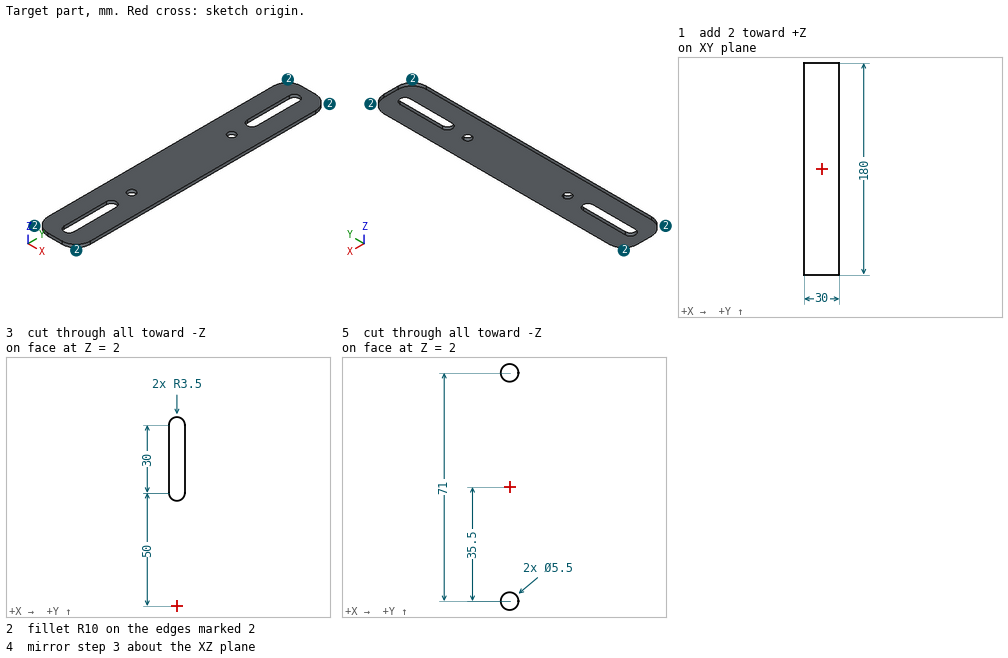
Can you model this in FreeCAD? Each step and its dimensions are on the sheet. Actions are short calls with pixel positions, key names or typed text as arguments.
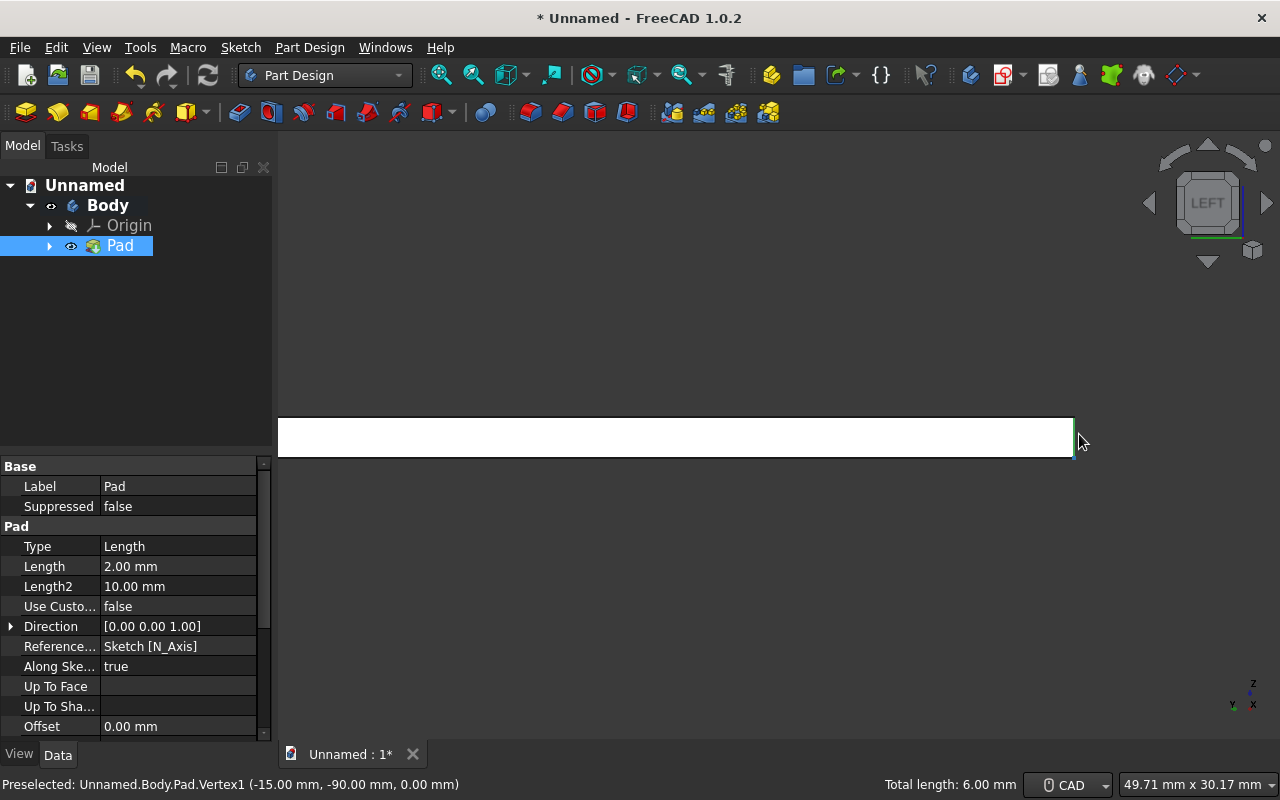
key(v)
key(f)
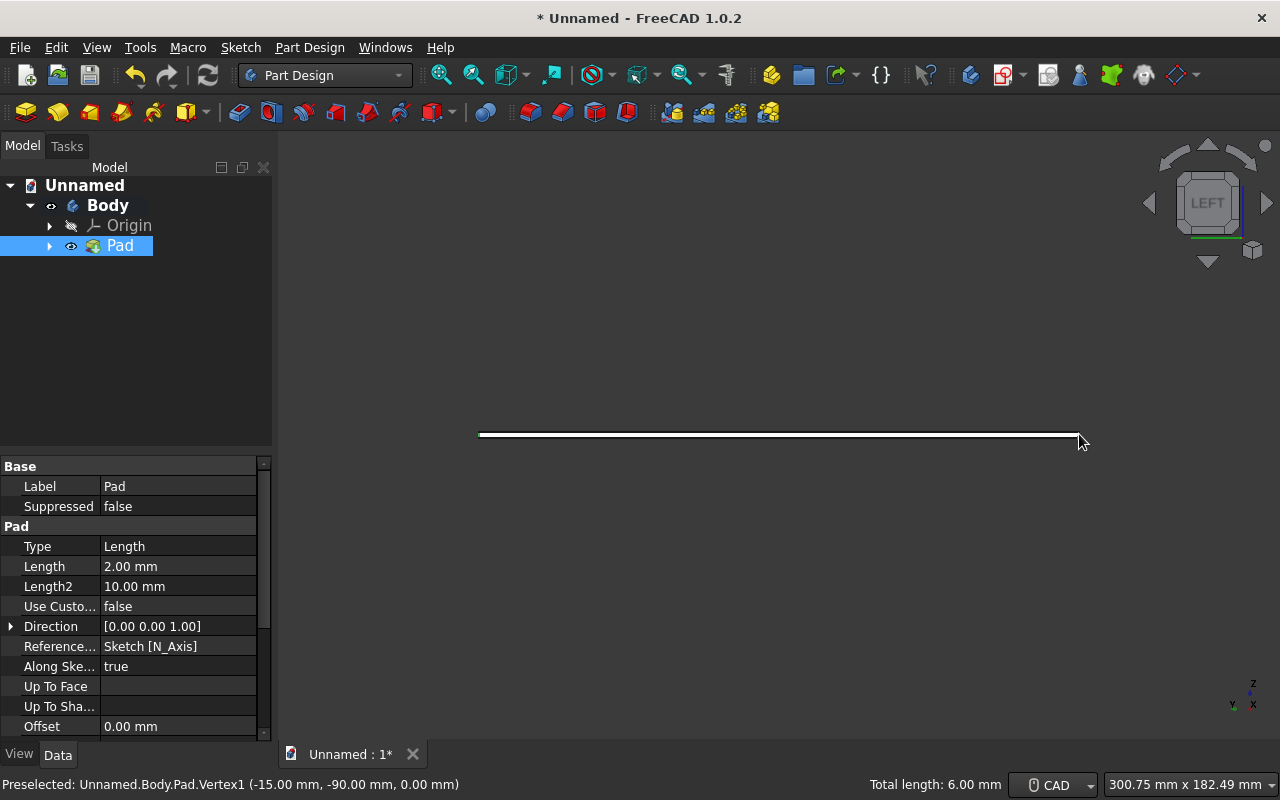
key(v)
key(3)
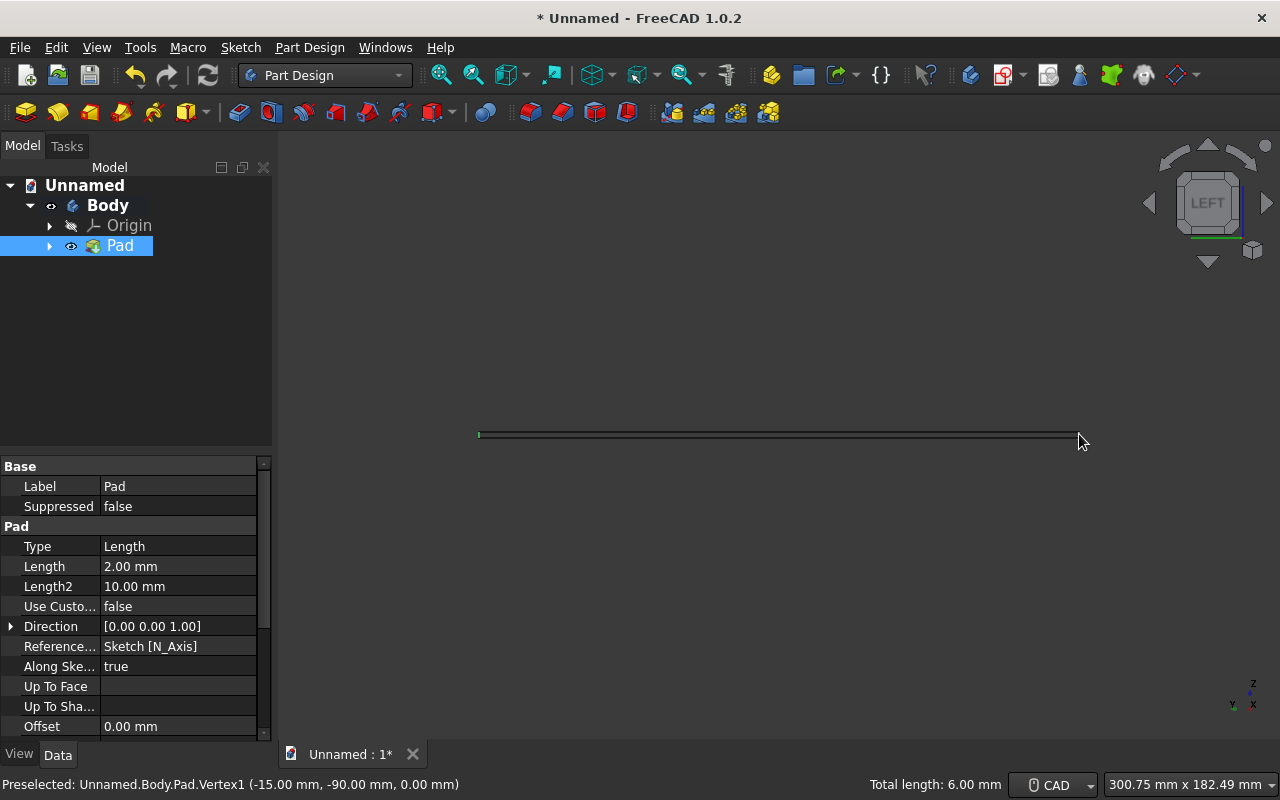
key(0)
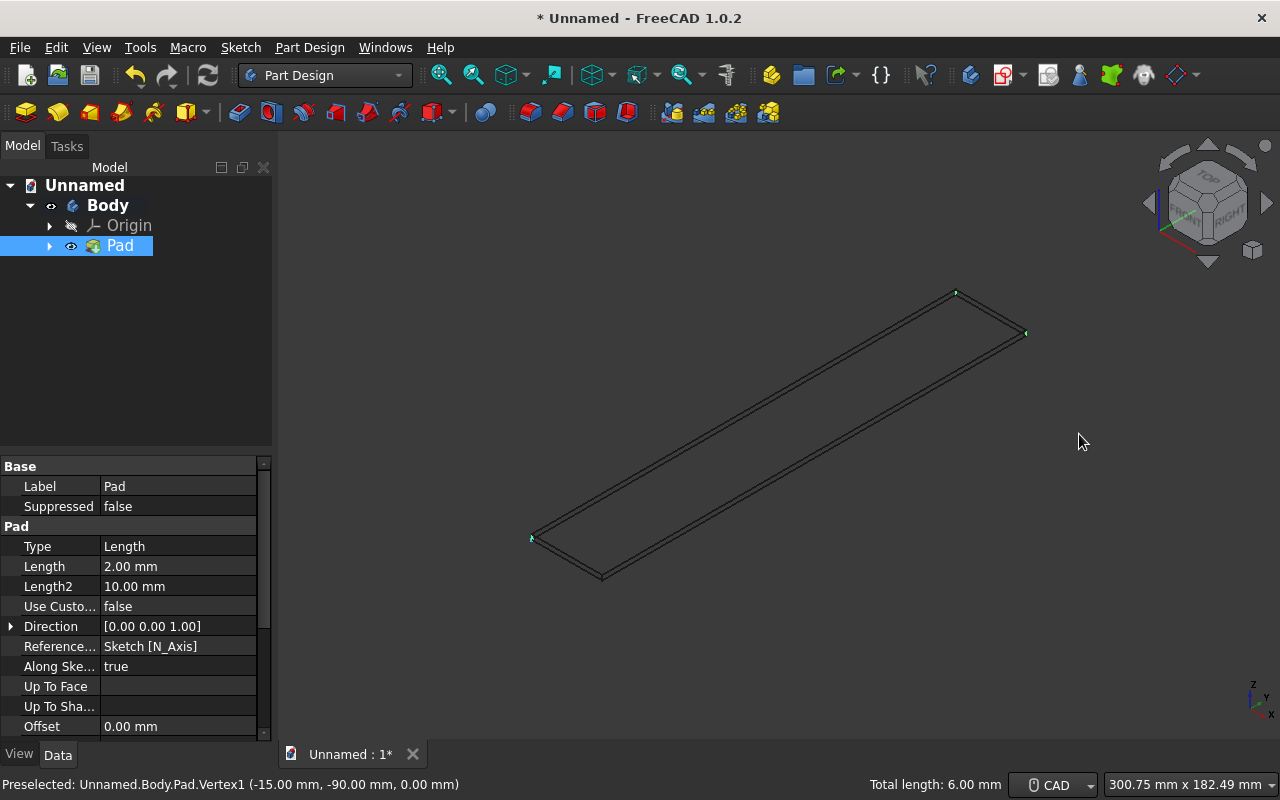
scroll(602, 577, up, 9)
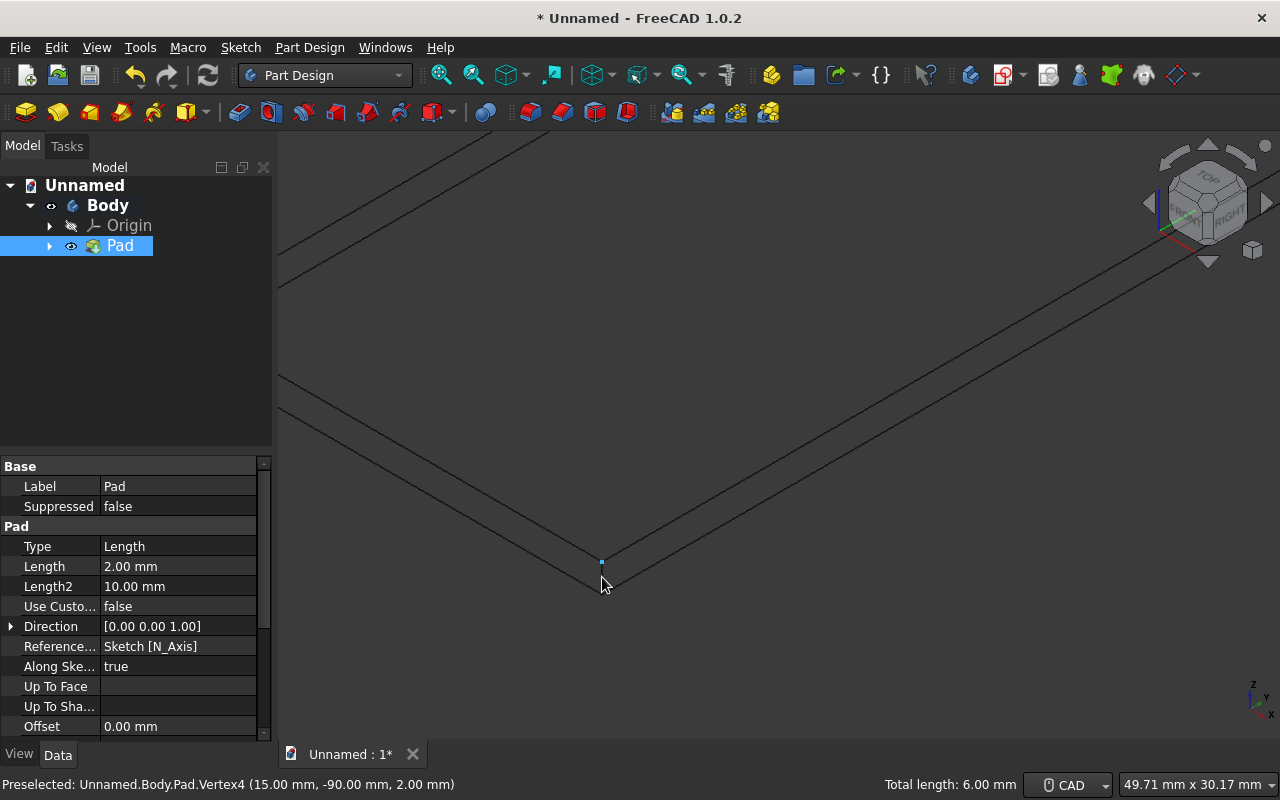
click(602, 577, ctrl)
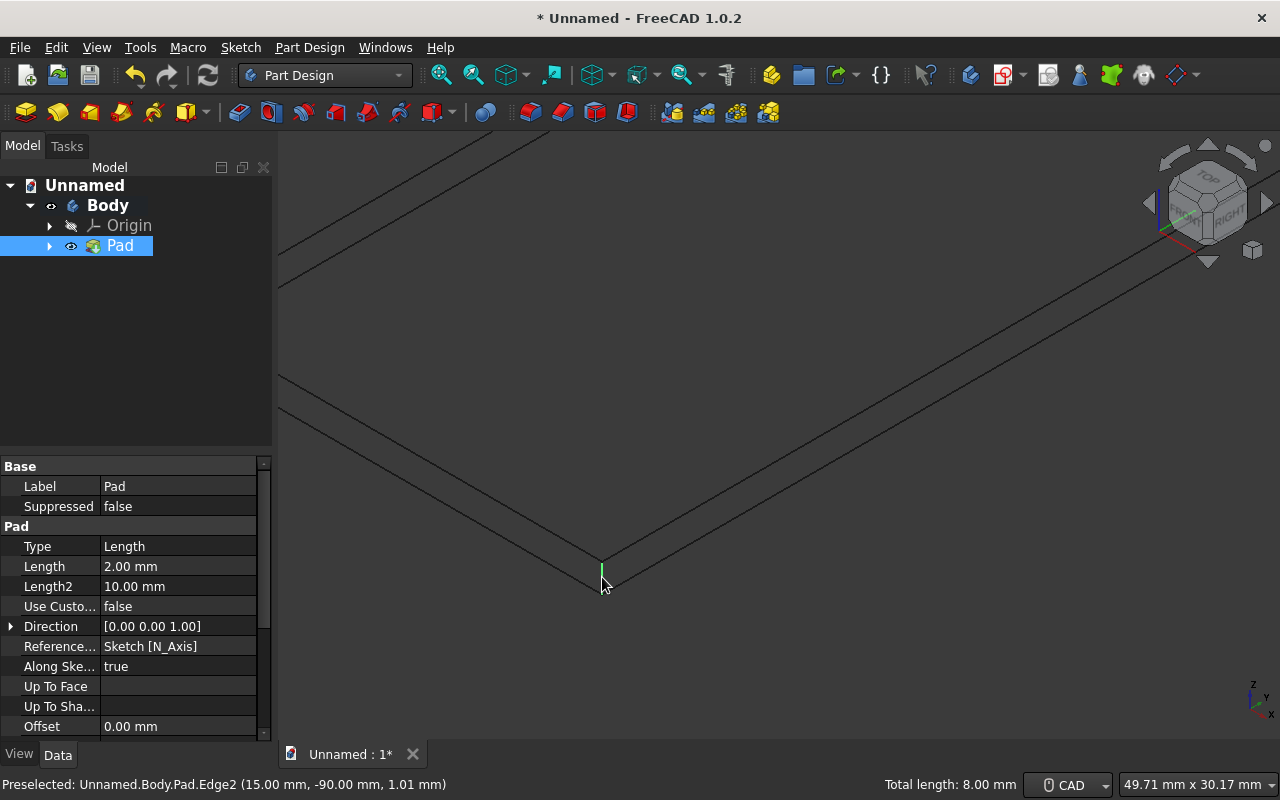
key(v)
key(1)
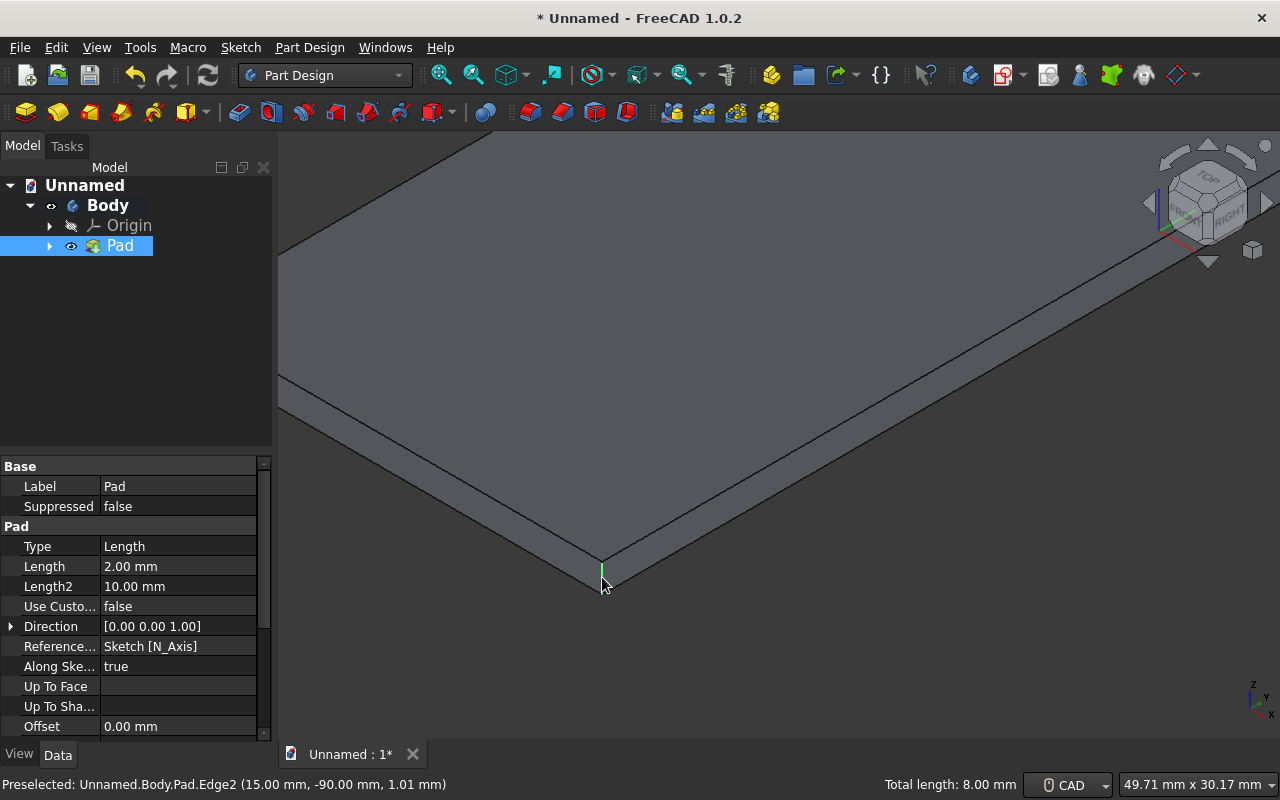
click(532, 112)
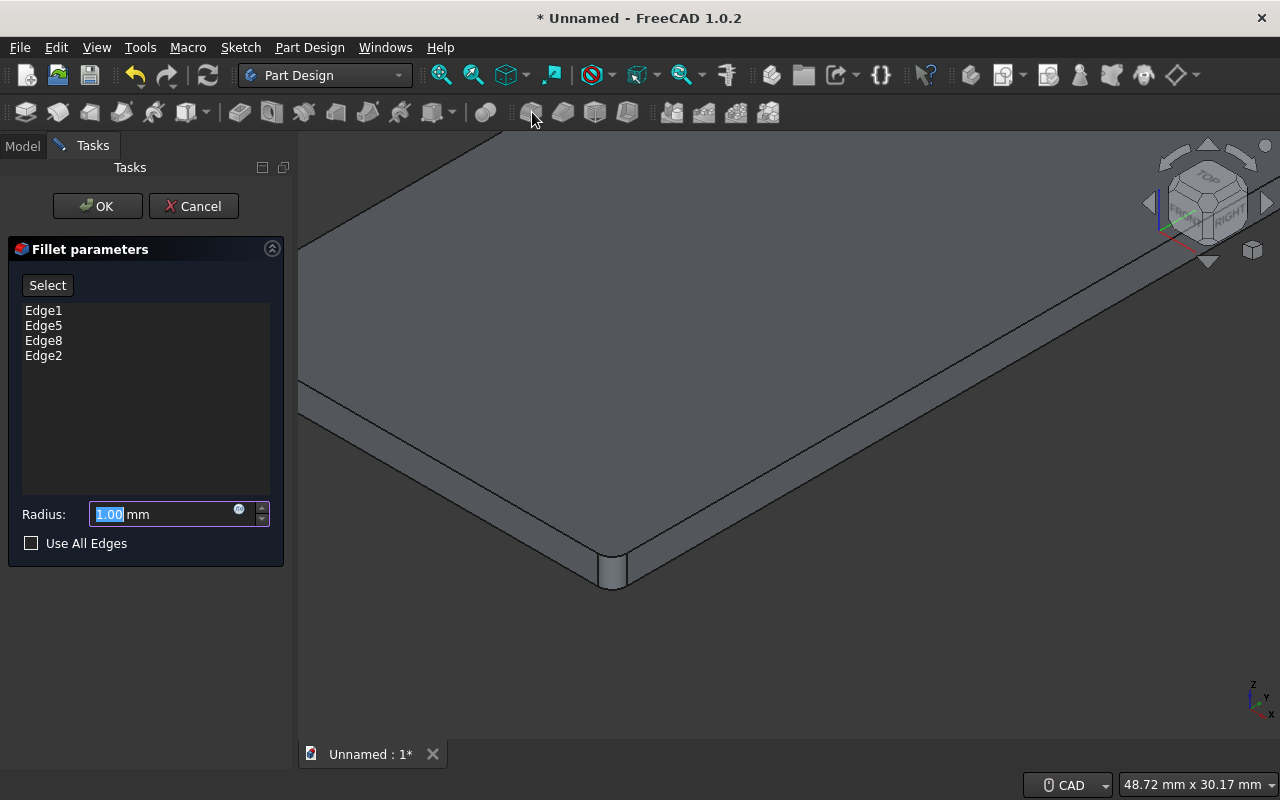
text(10)
key(Tab)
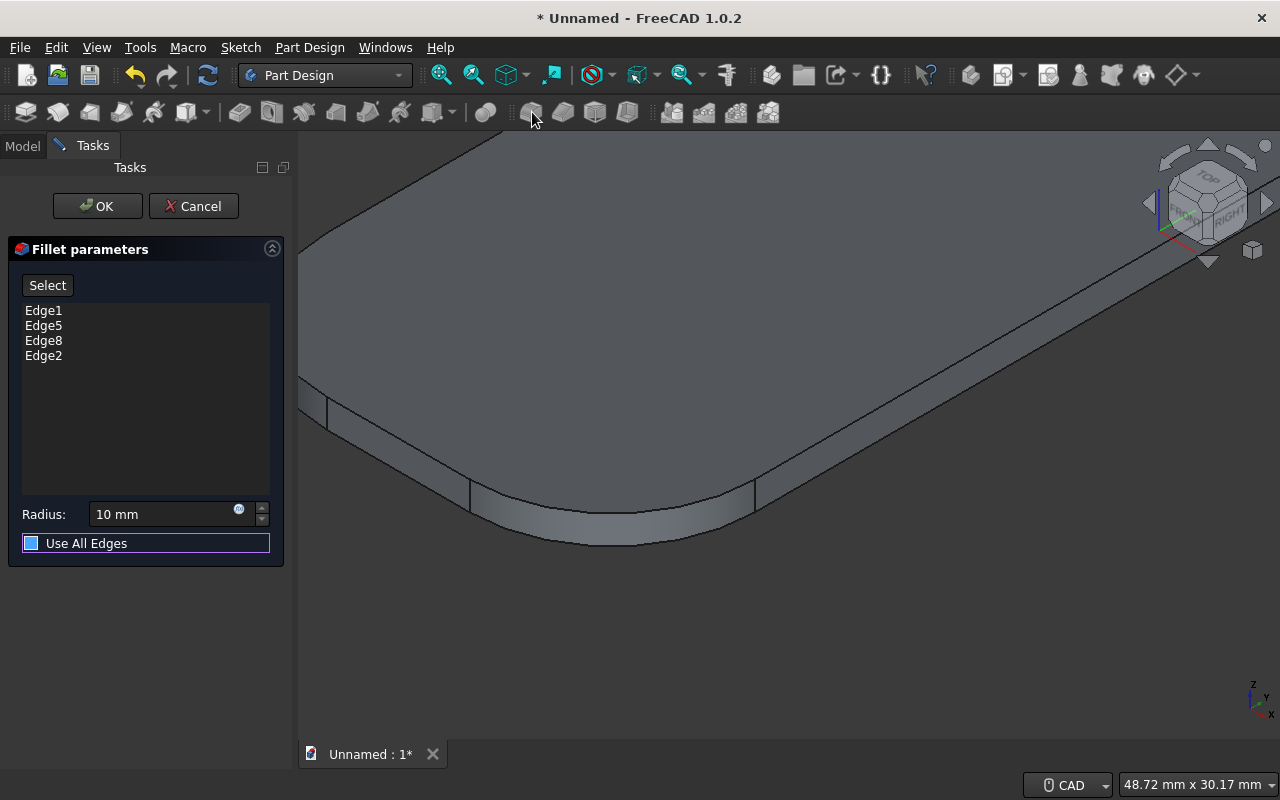
click(98, 206)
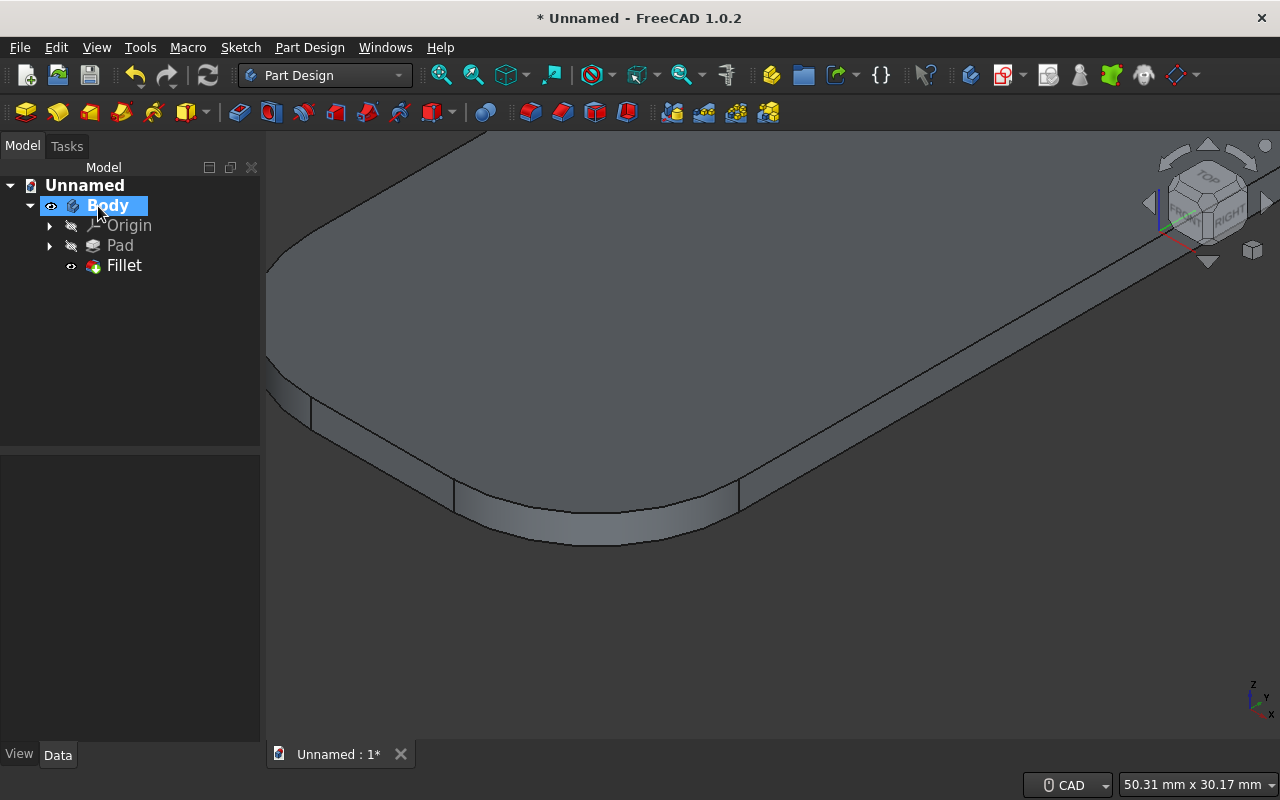
click(442, 76)